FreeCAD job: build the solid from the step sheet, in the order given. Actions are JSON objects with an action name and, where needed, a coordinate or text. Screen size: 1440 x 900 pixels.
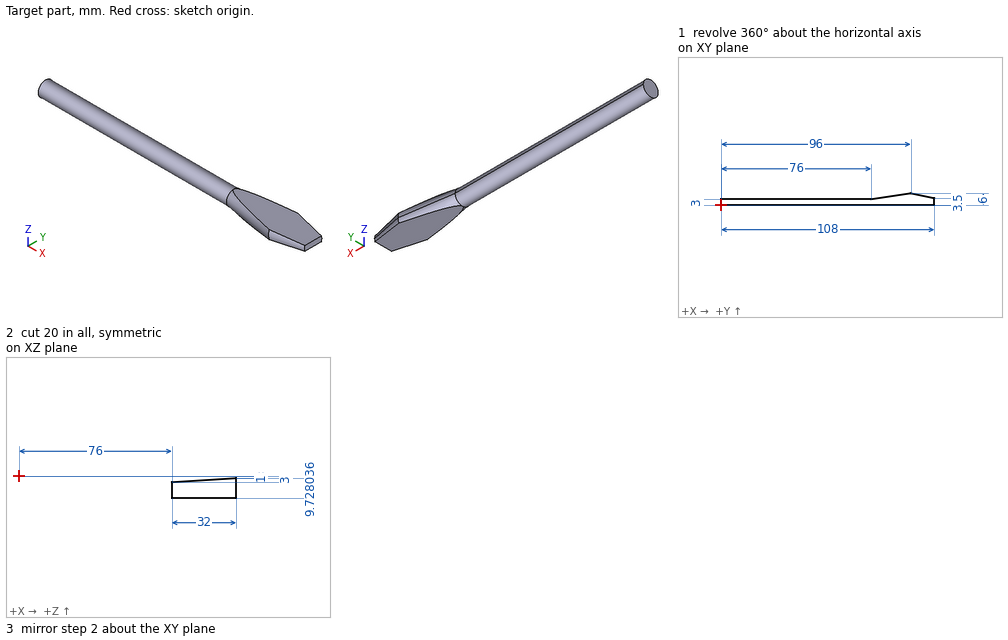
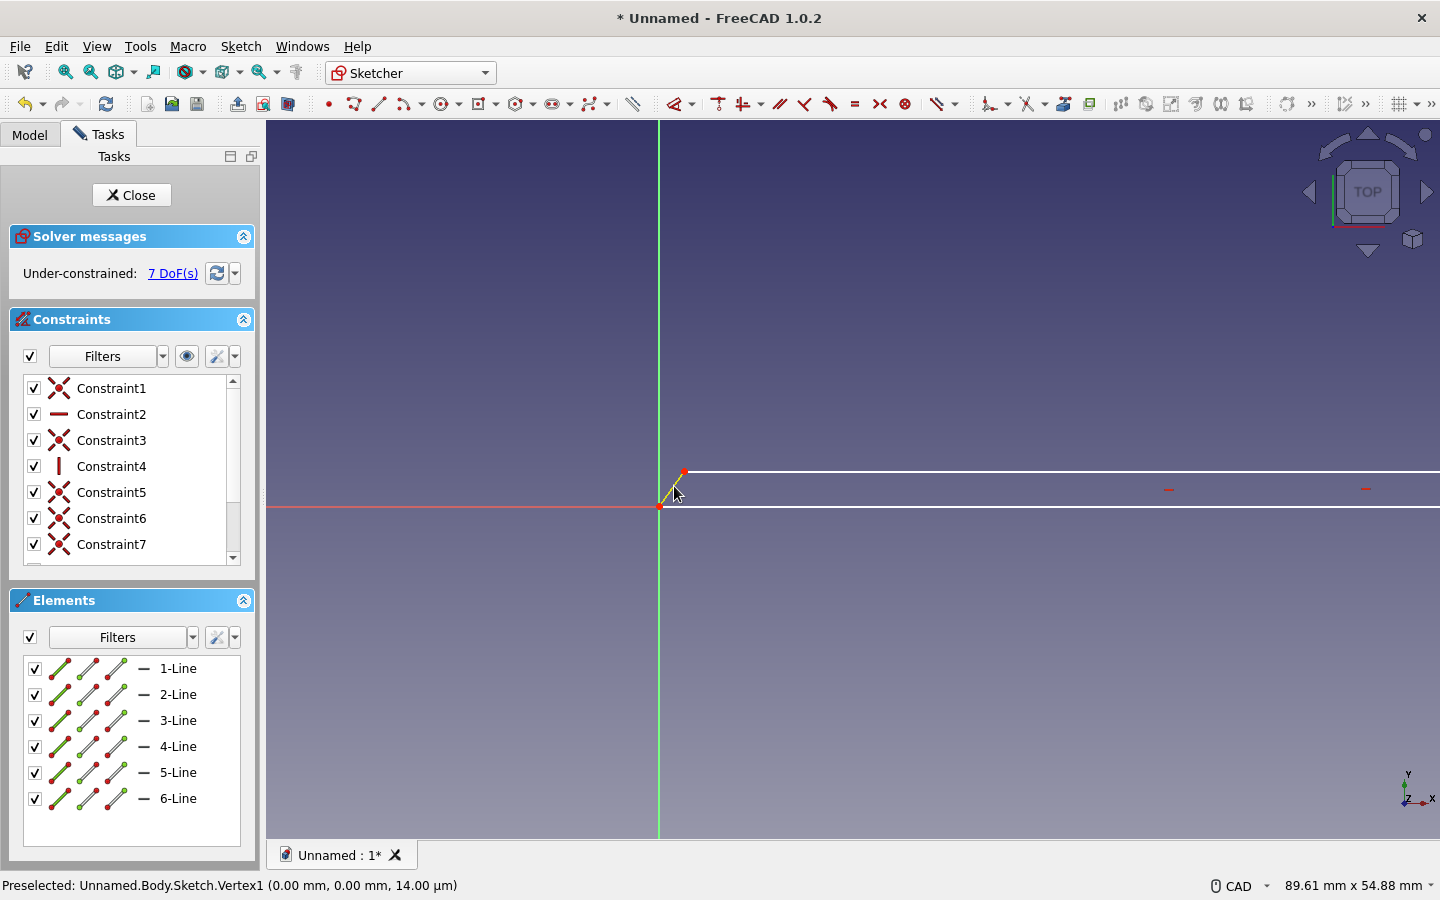
{"action": "left_click", "coordinate": [674, 486]}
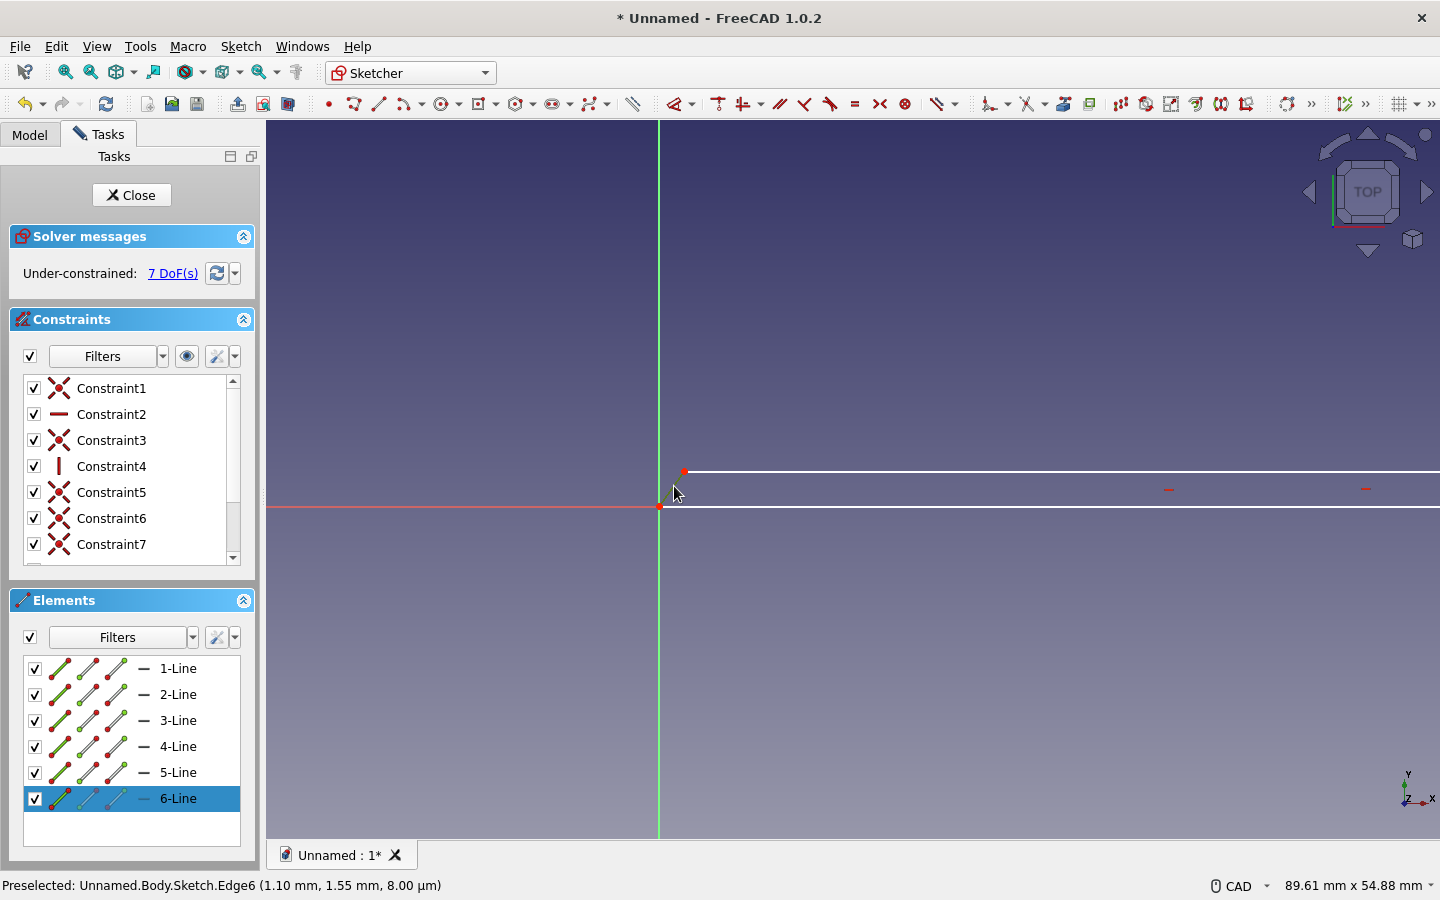
{"action": "key", "text": "v"}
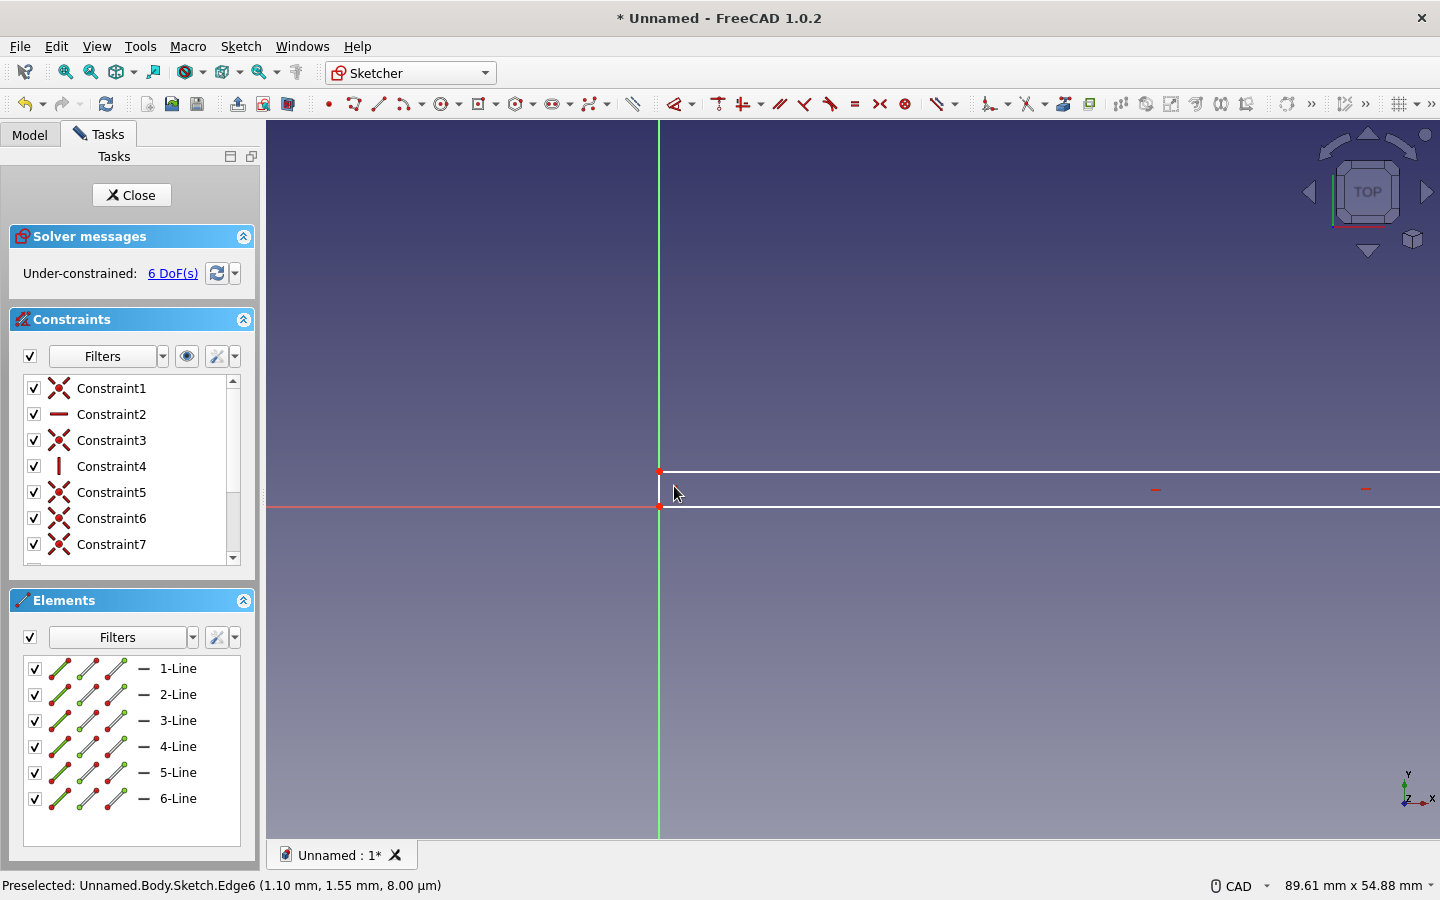
{"action": "scroll", "coordinate": [659, 482], "scroll_direction": "up", "scroll_amount": 2}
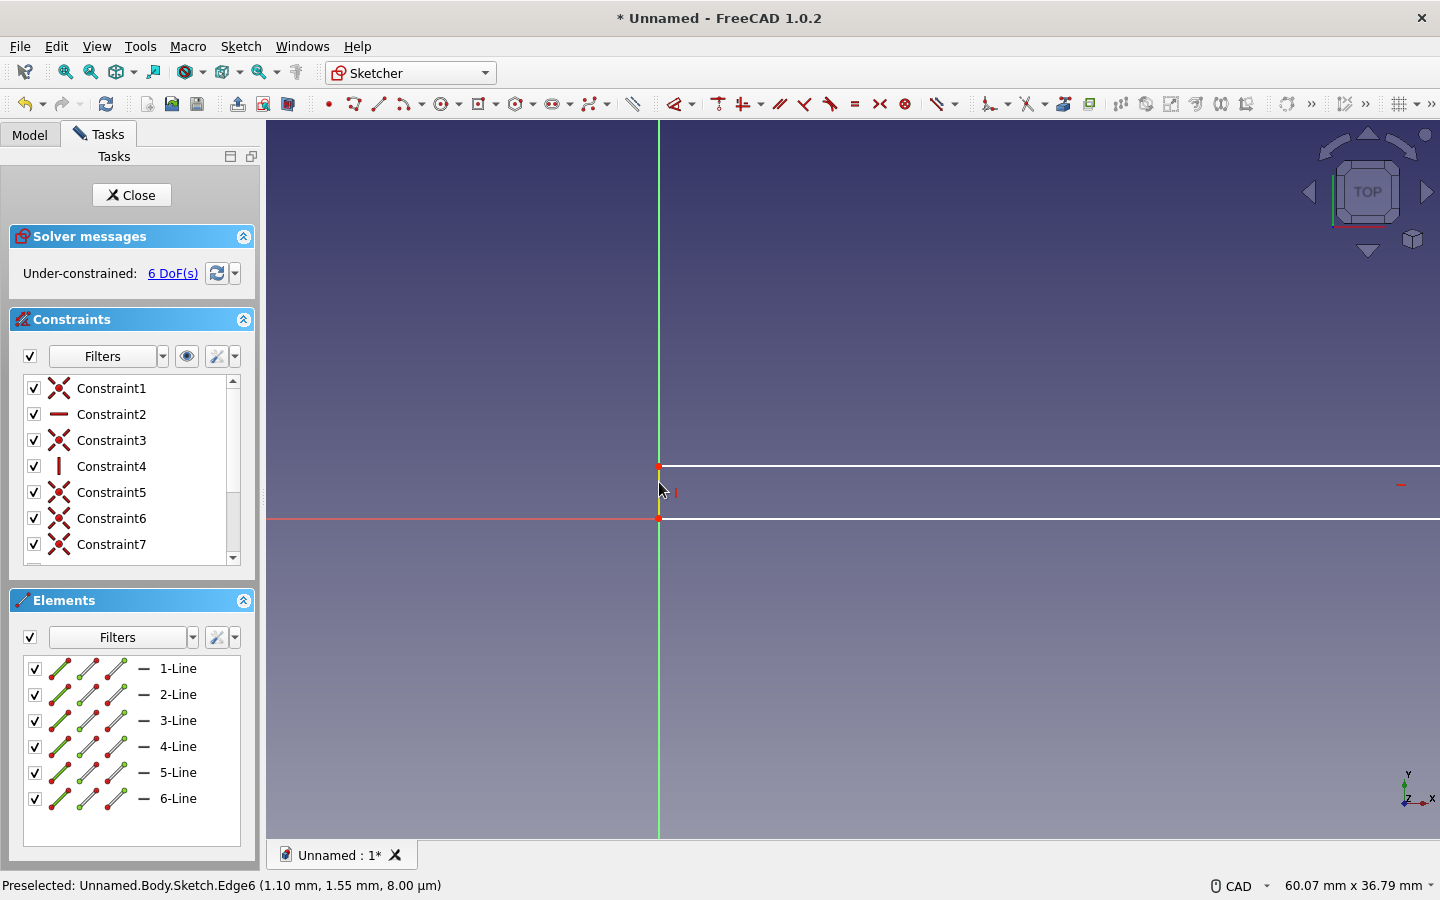
{"action": "left_click", "coordinate": [659, 482]}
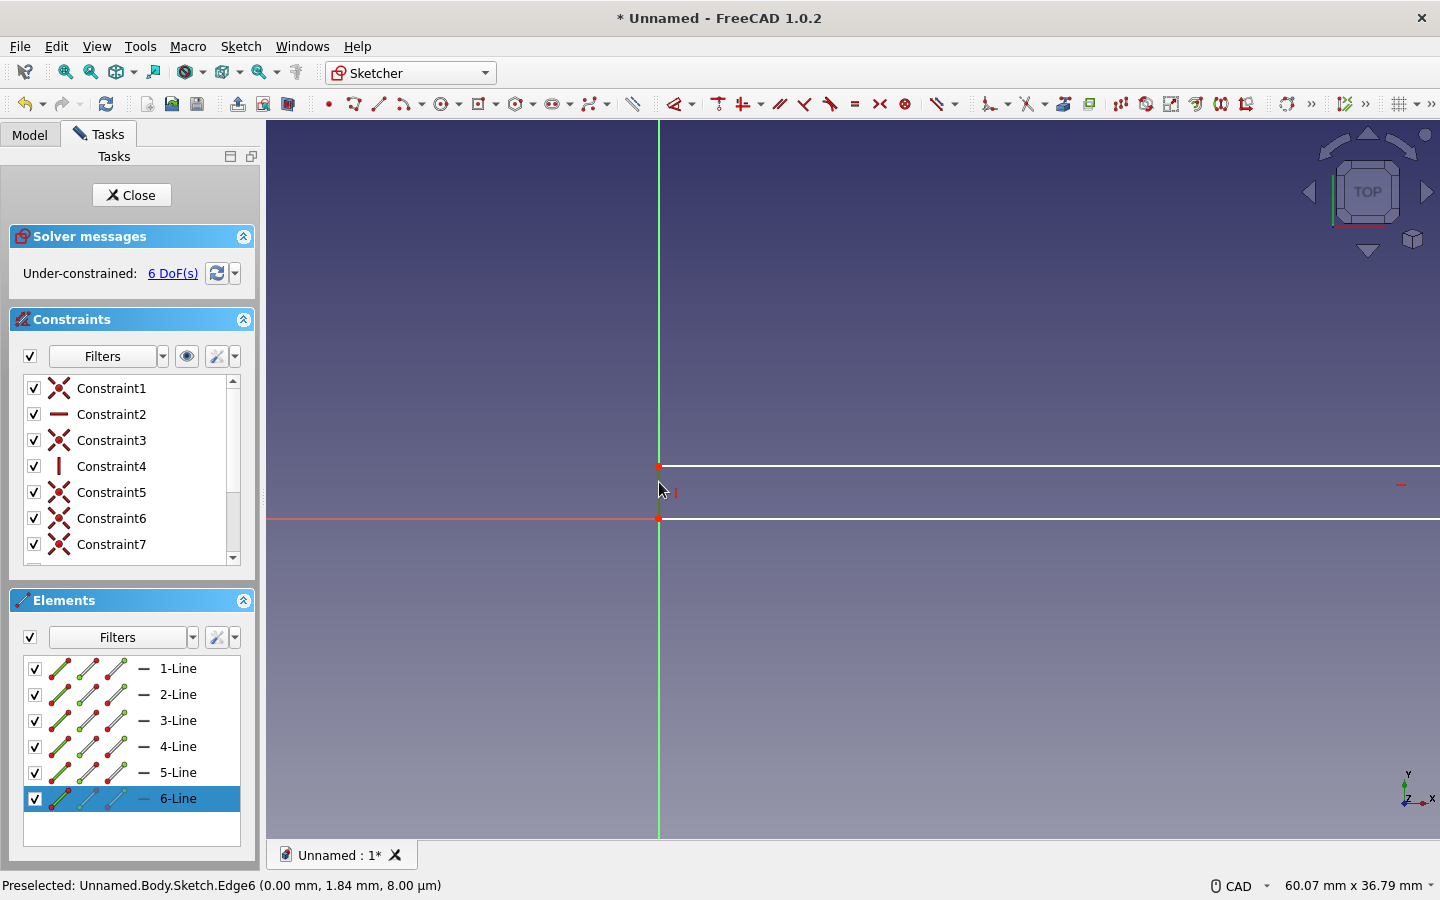
{"action": "key", "text": "i"}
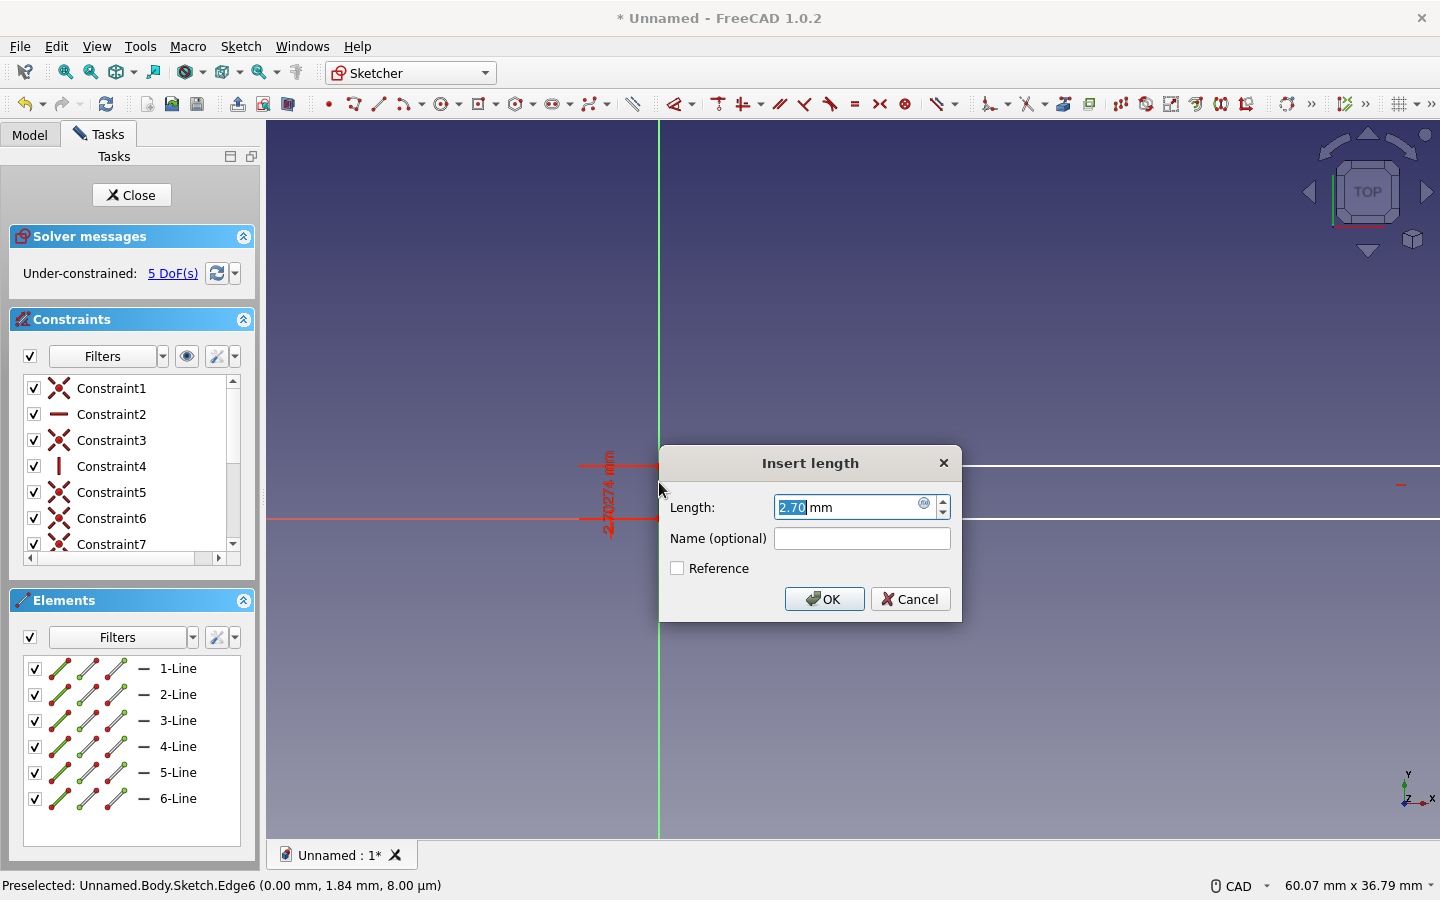
{"action": "type", "text": "3"}
{"action": "key", "text": "Return"}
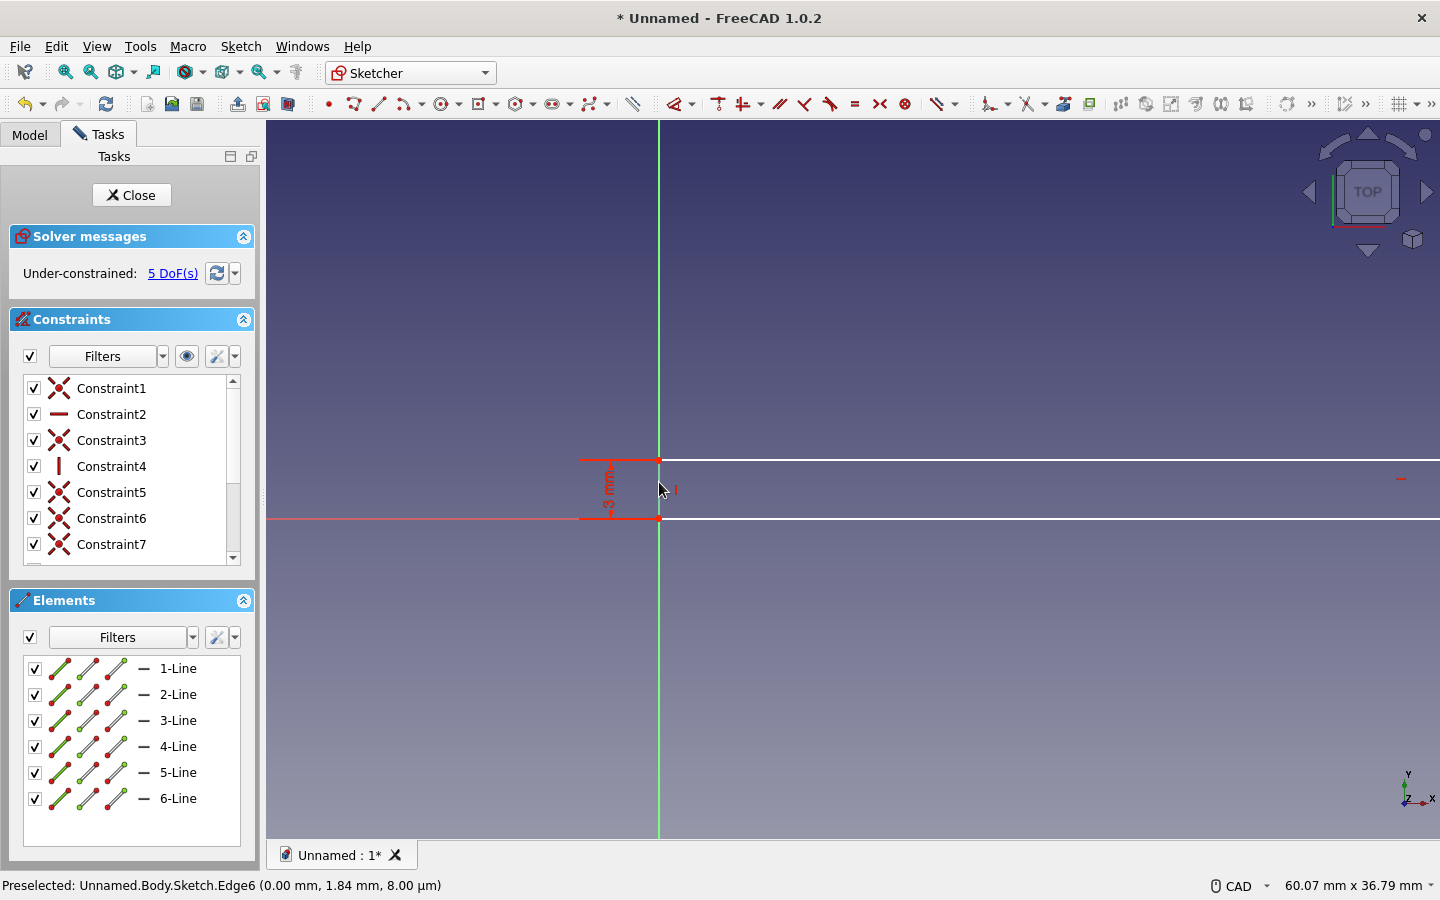
{"action": "scroll", "coordinate": [384, 488], "scroll_direction": "down", "scroll_amount": 6}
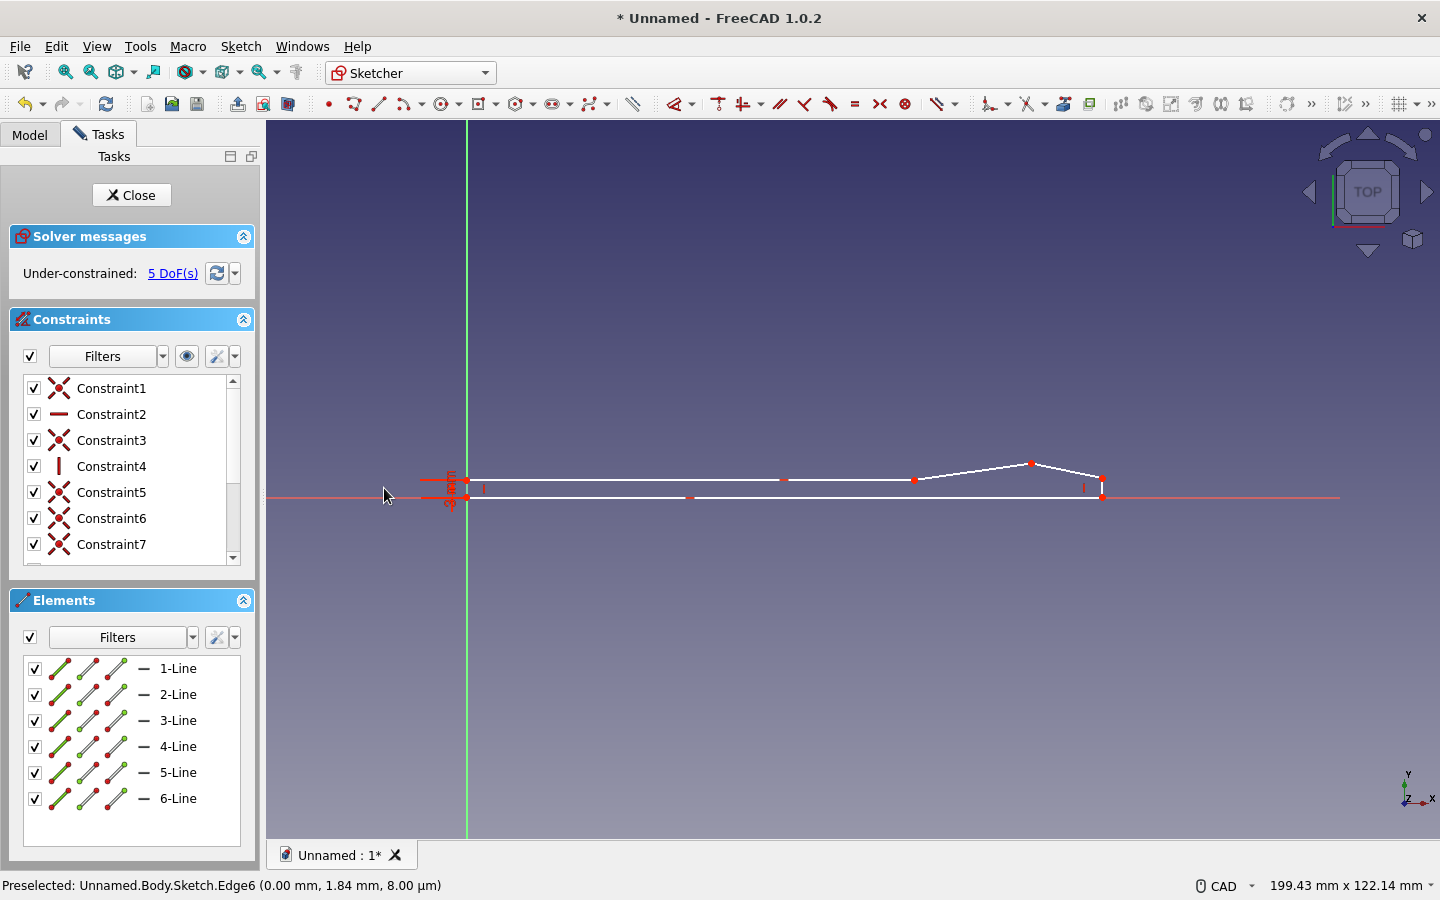
{"action": "left_click", "coordinate": [601, 480]}